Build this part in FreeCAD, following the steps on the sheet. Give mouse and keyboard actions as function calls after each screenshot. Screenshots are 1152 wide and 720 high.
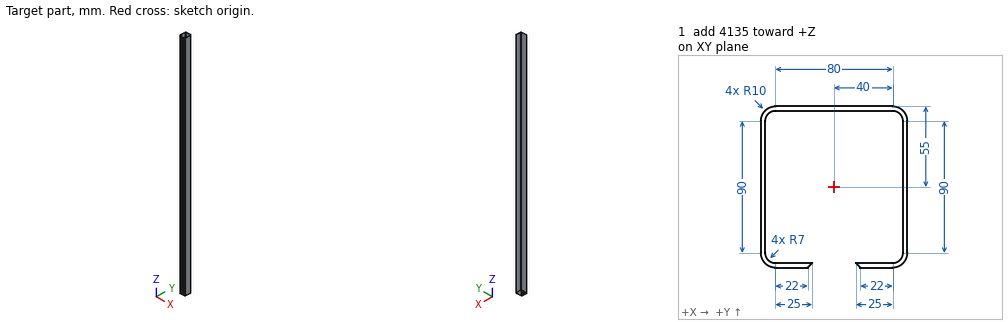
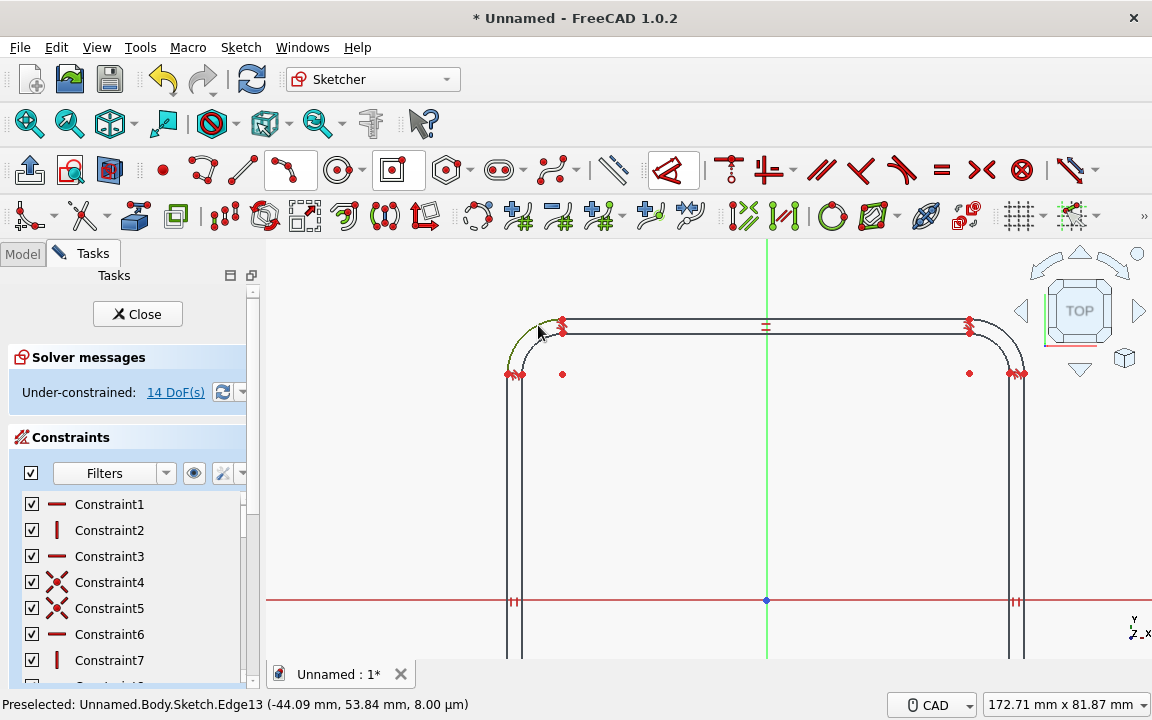
scroll(537, 326, down, 4)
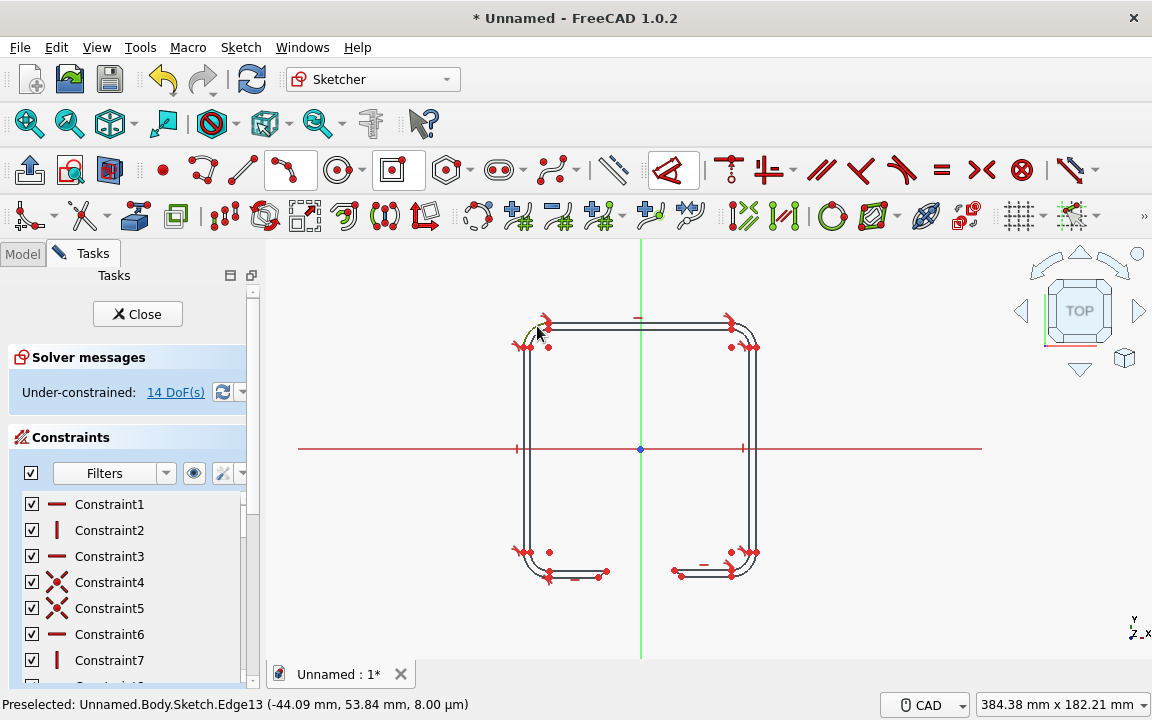
scroll(527, 564, up, 4)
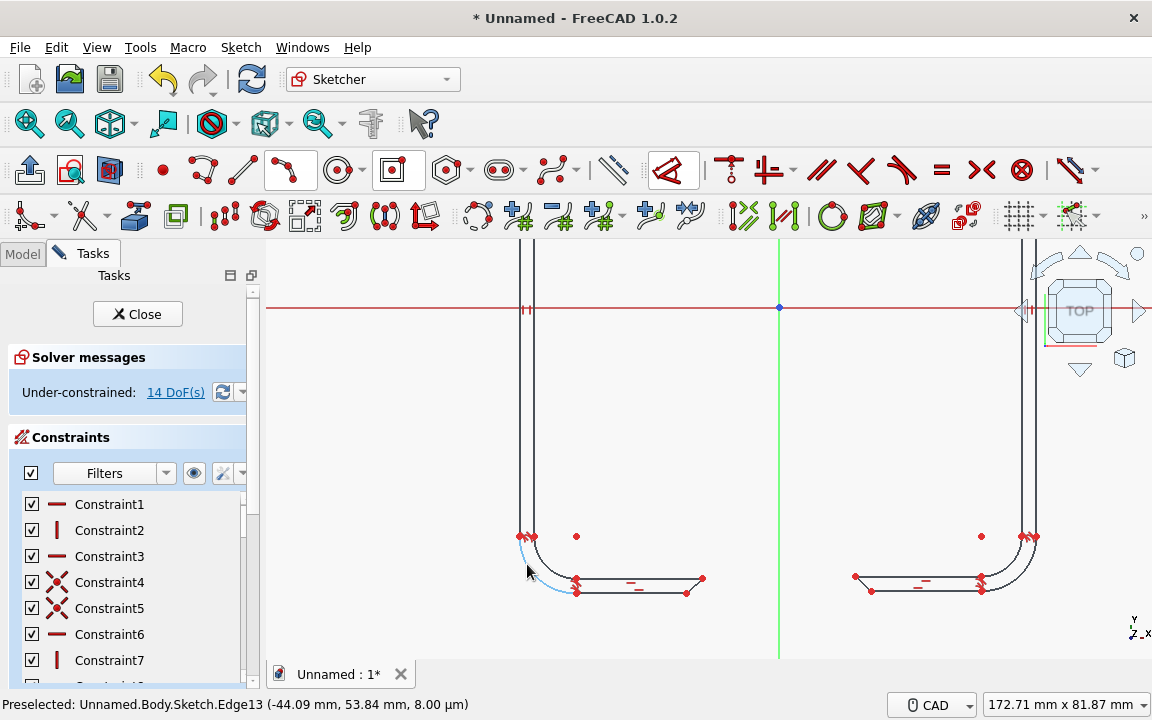
click(526, 563)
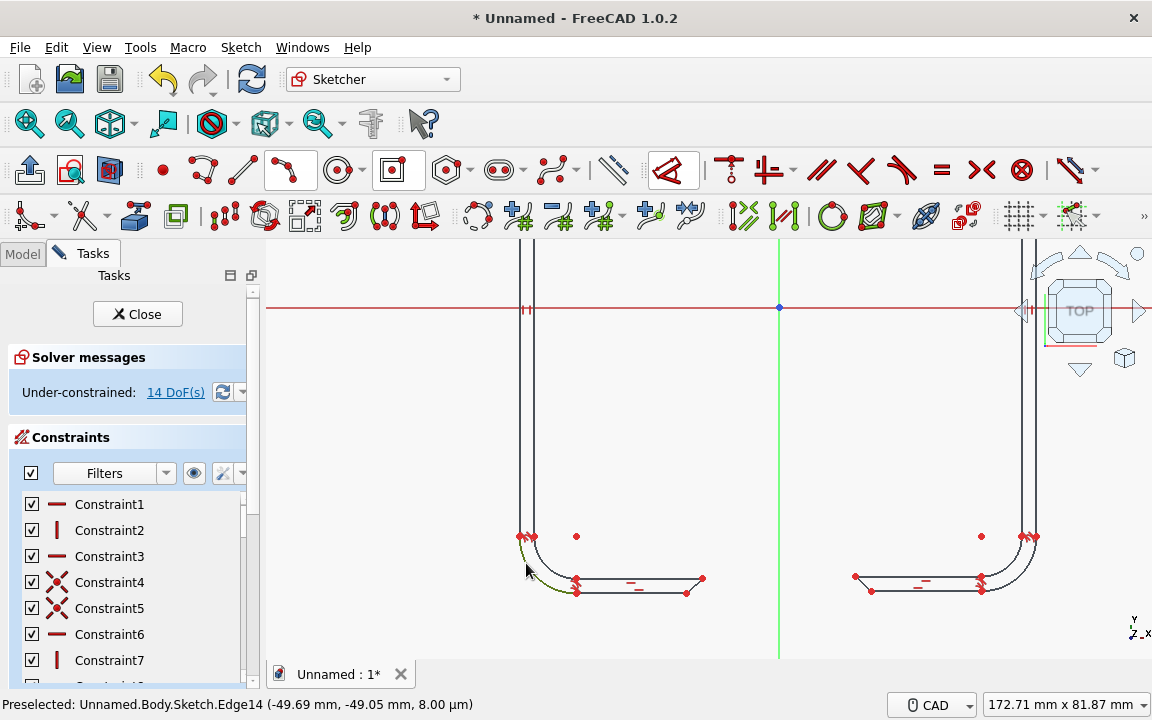
scroll(527, 564, down, 4)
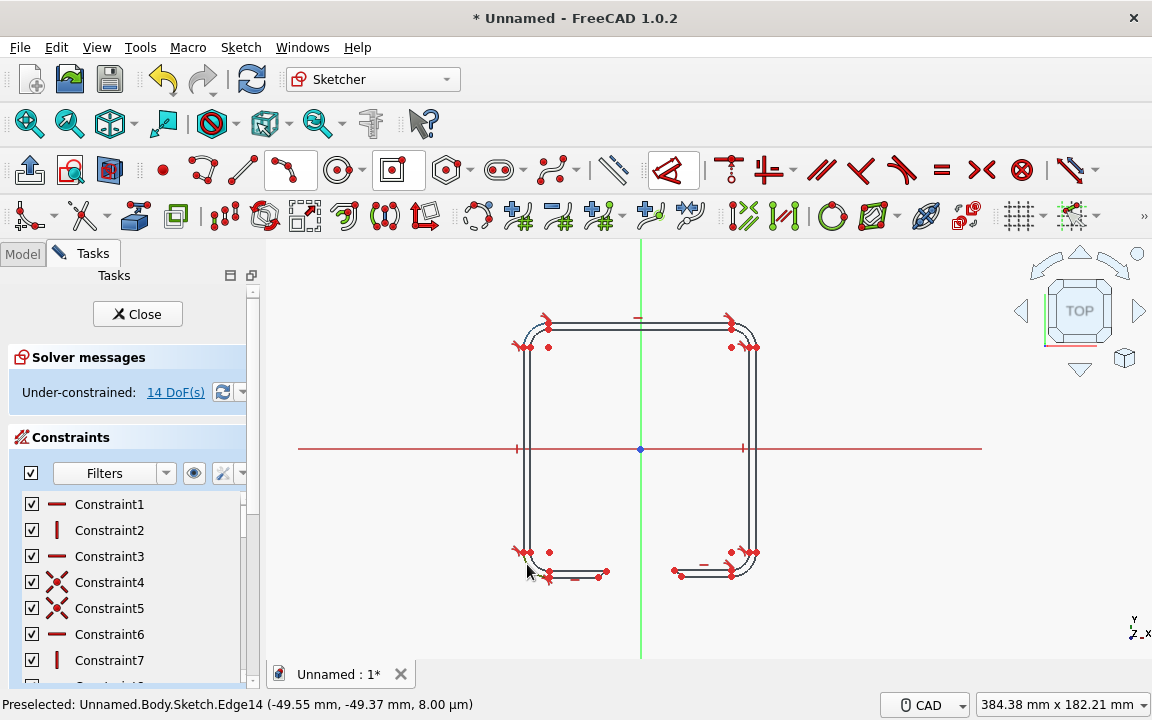
scroll(743, 574, up, 4)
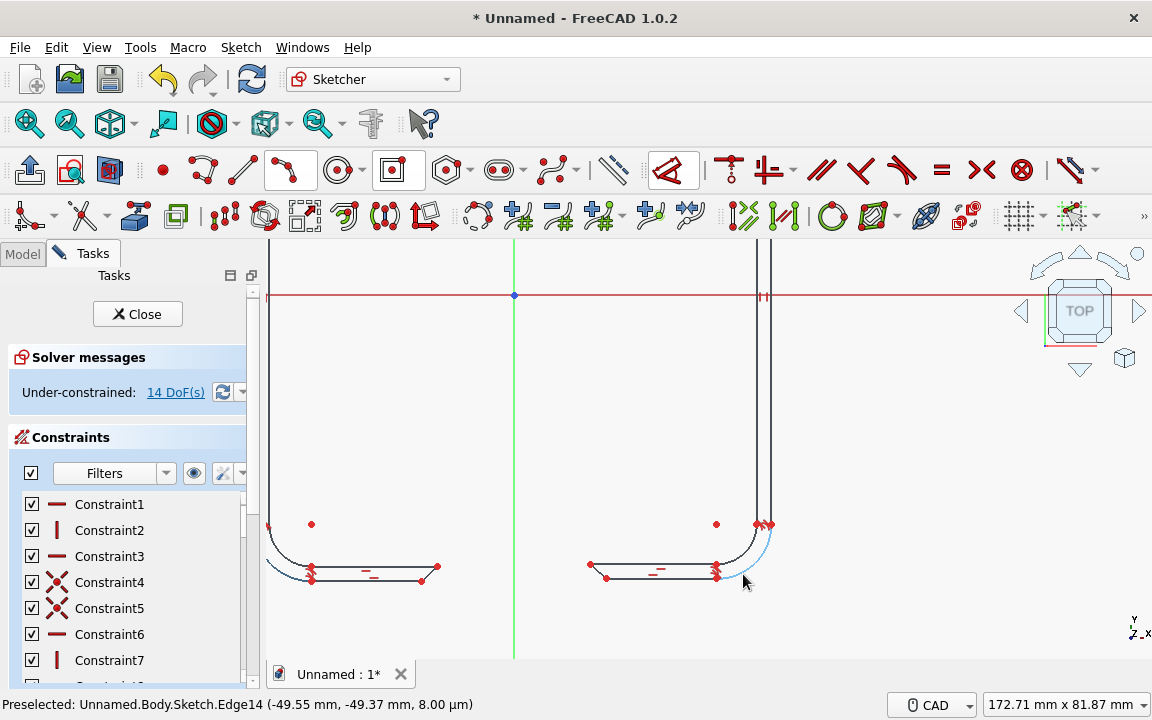
click(742, 573)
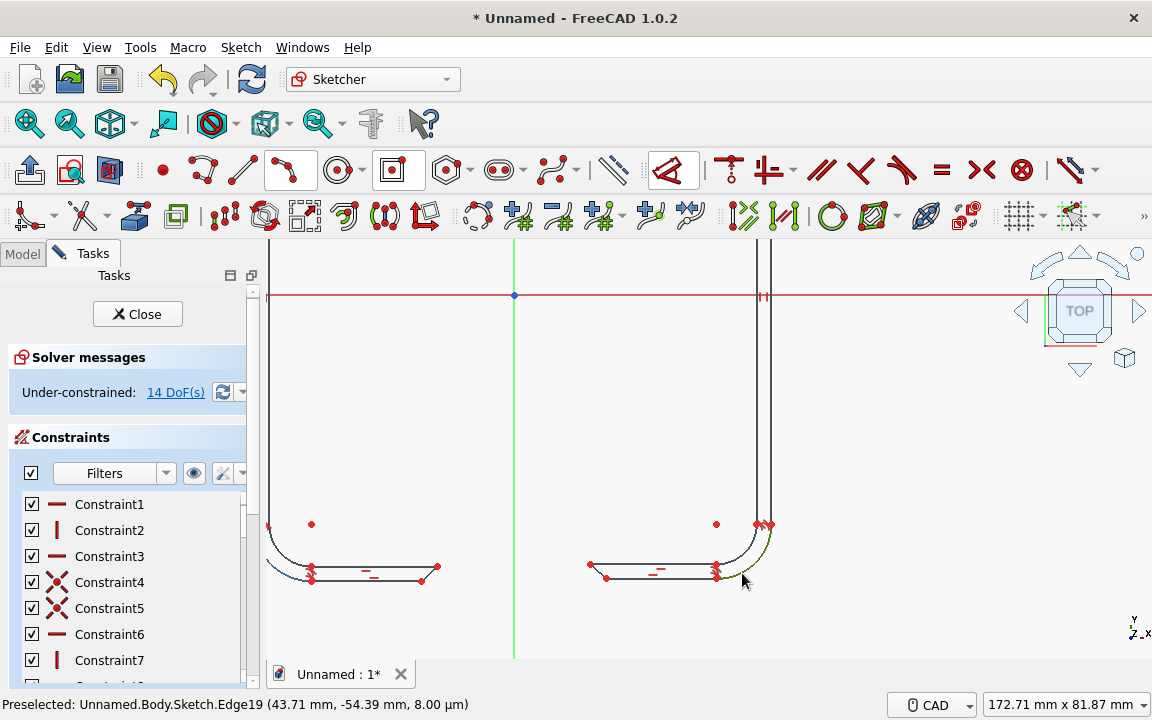
scroll(744, 574, down, 4)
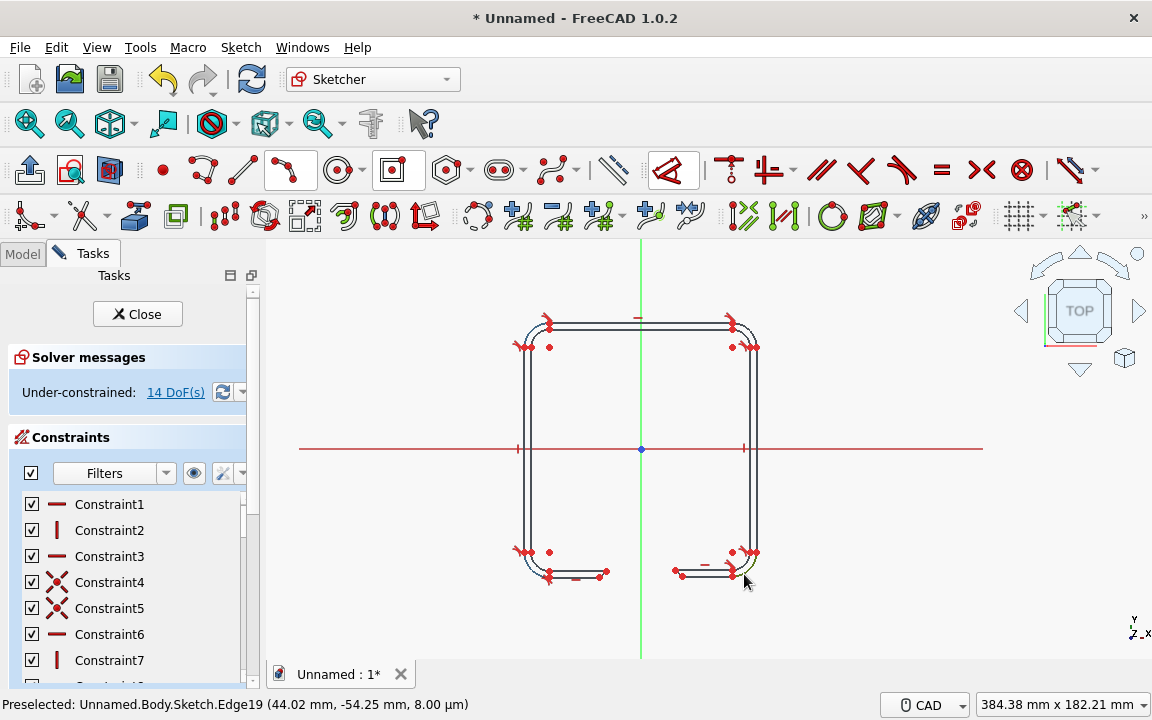
scroll(754, 336, up, 4)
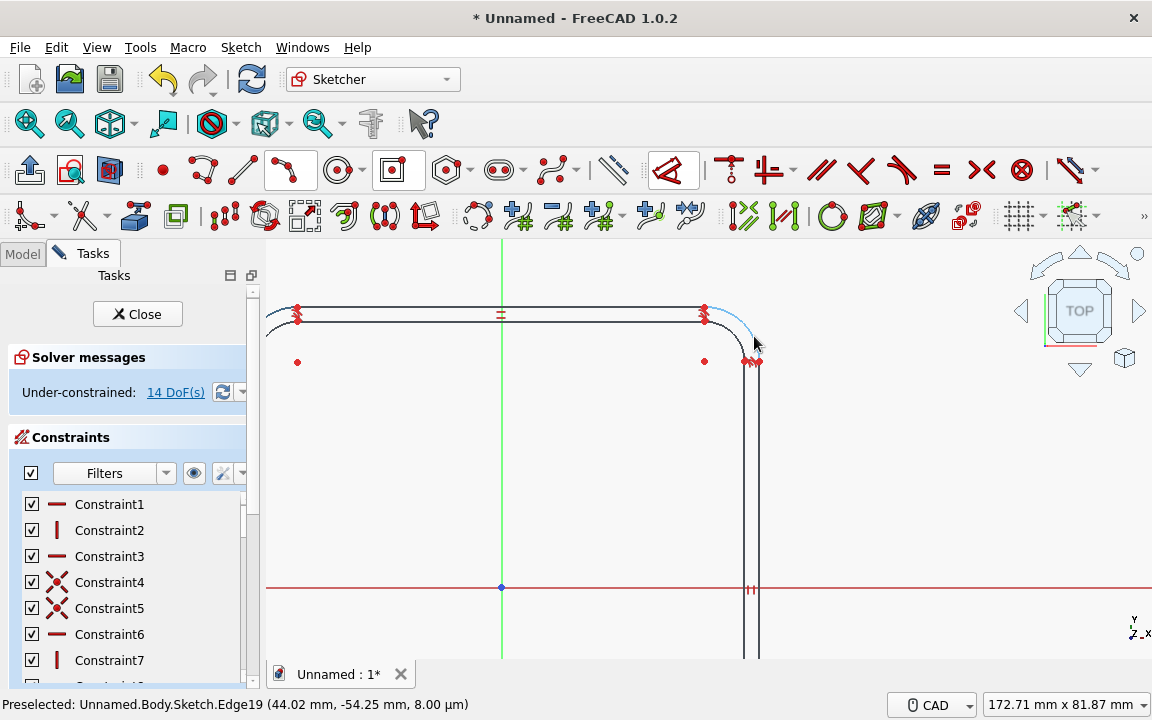
click(753, 337)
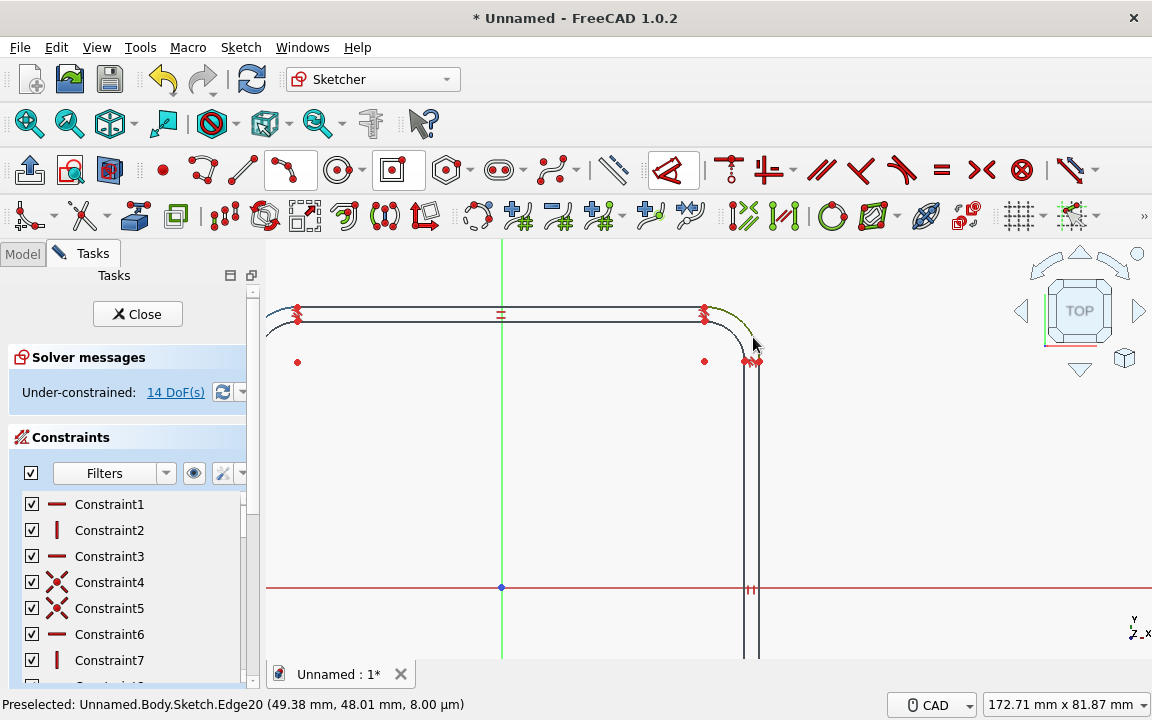
click(942, 170)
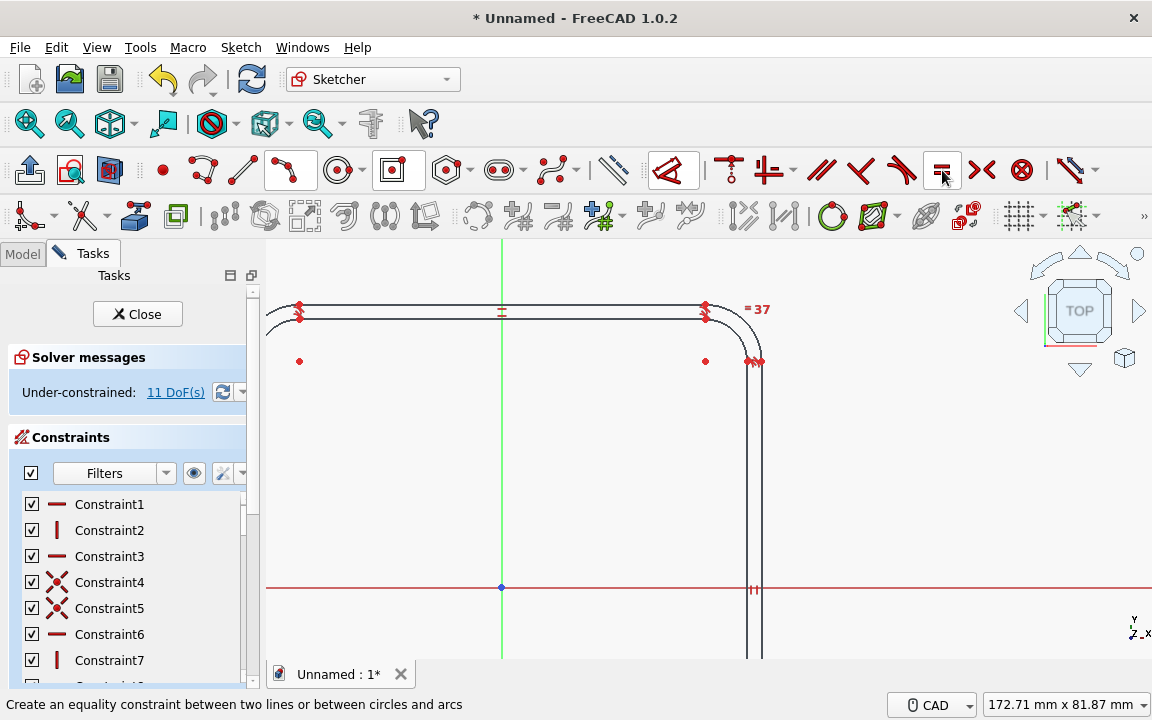
click(668, 170)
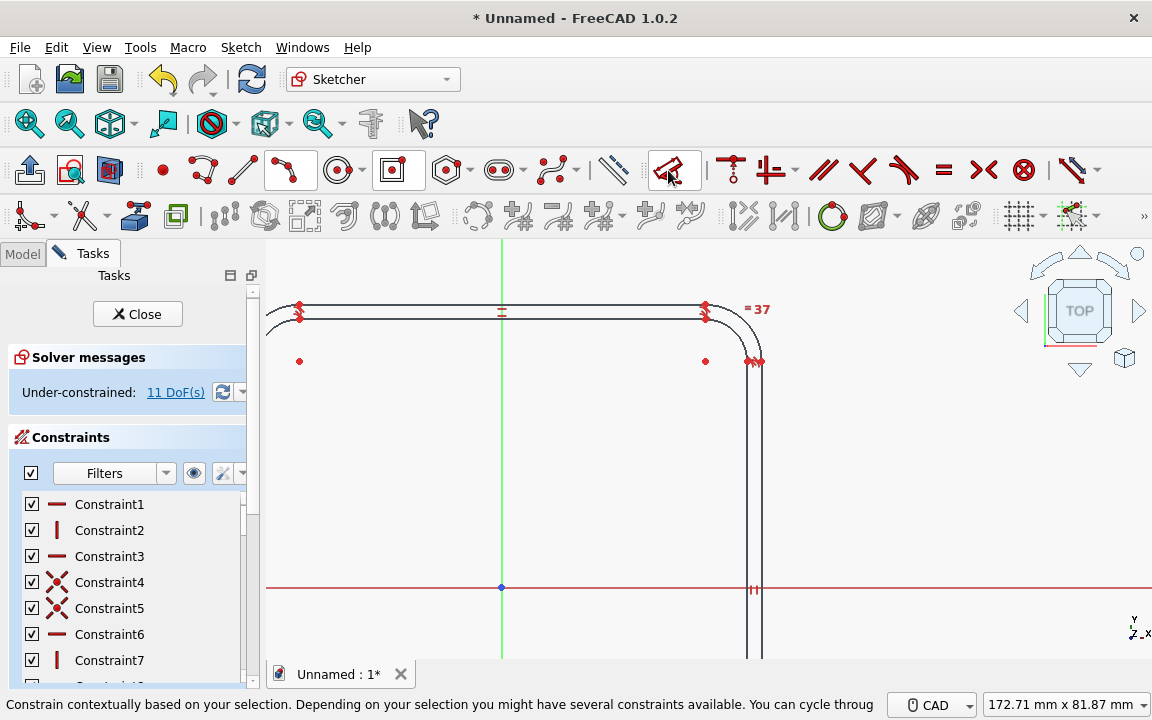
scroll(754, 336, down, 4)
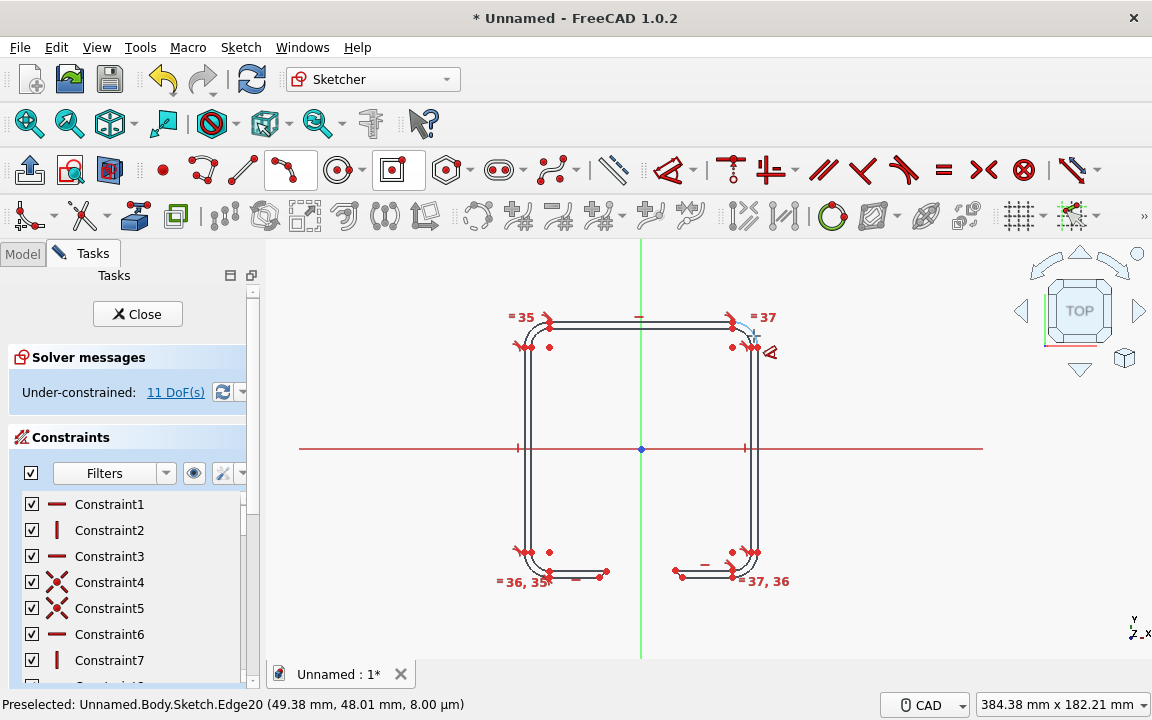
scroll(538, 325, up, 4)